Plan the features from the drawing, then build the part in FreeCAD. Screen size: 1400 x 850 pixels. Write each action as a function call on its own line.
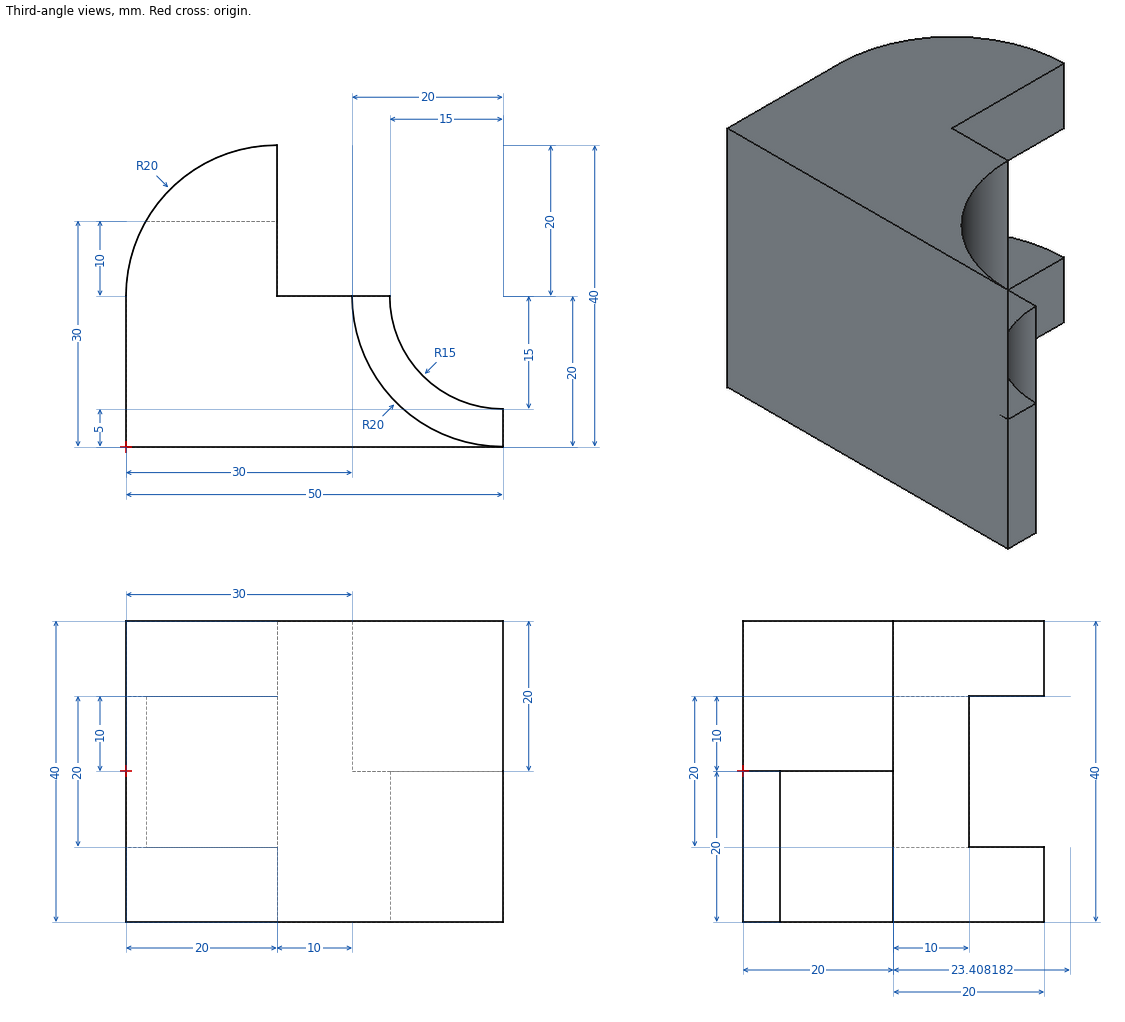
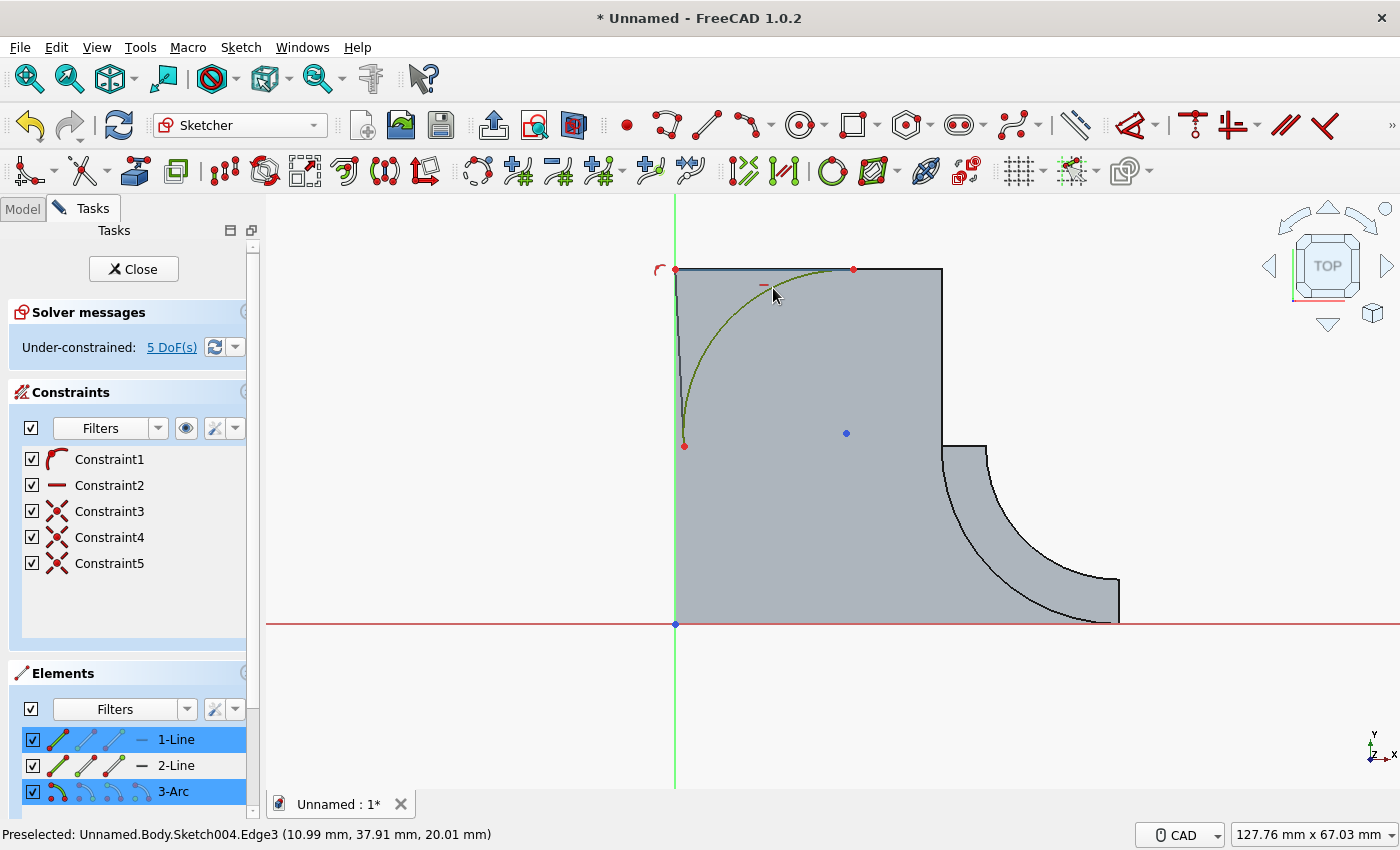
key(t)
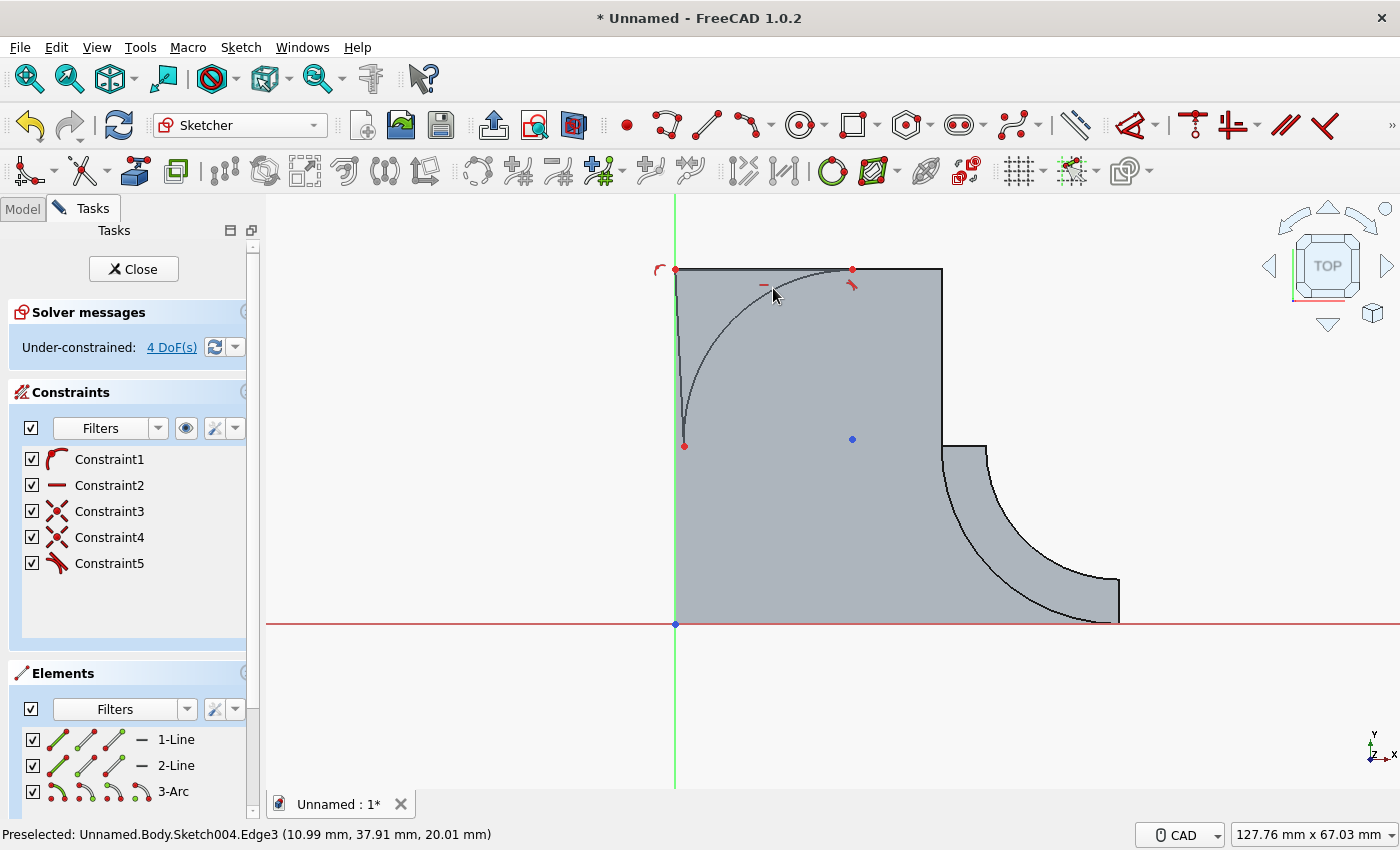
click(678, 323)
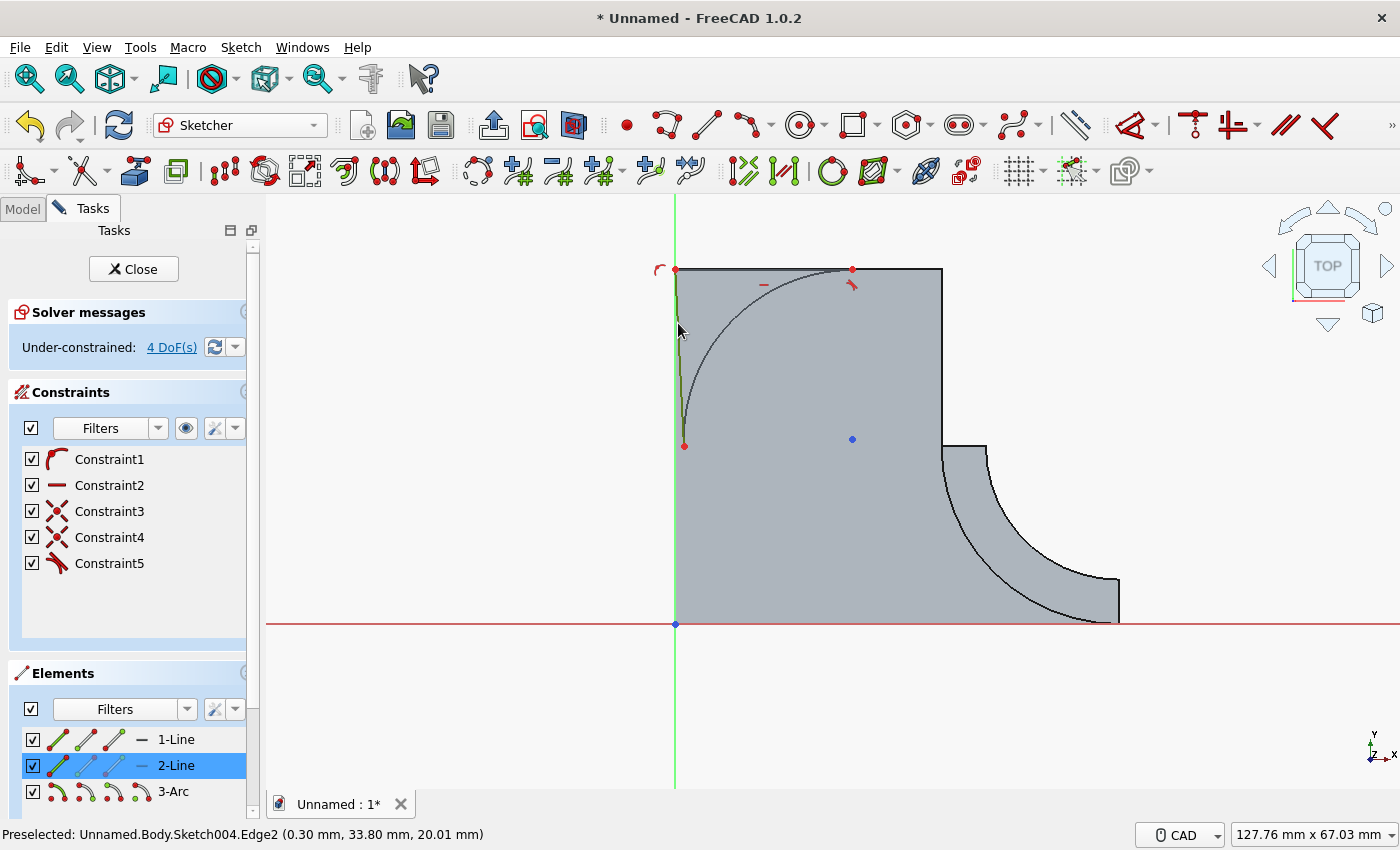
click(774, 290)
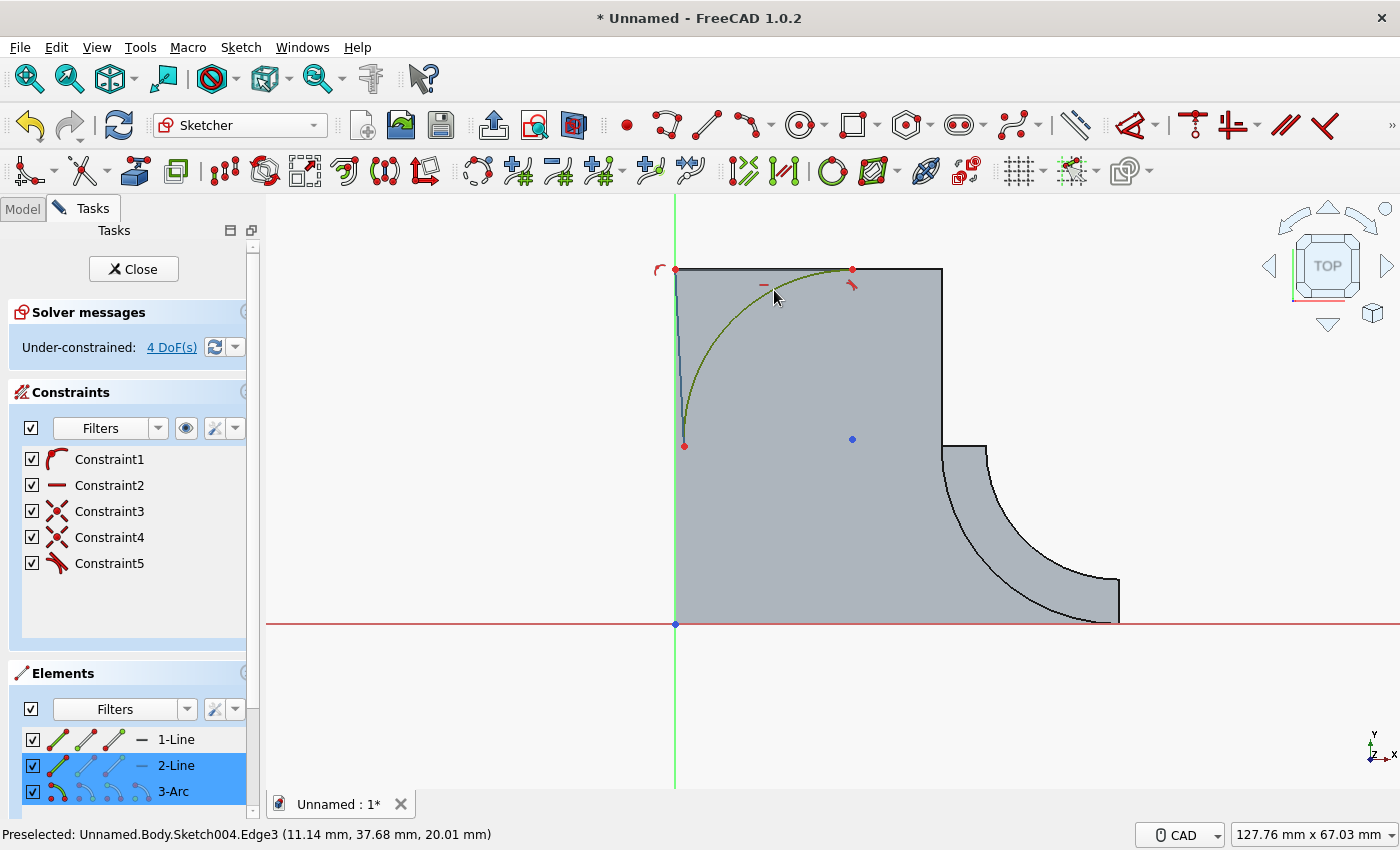
key(t)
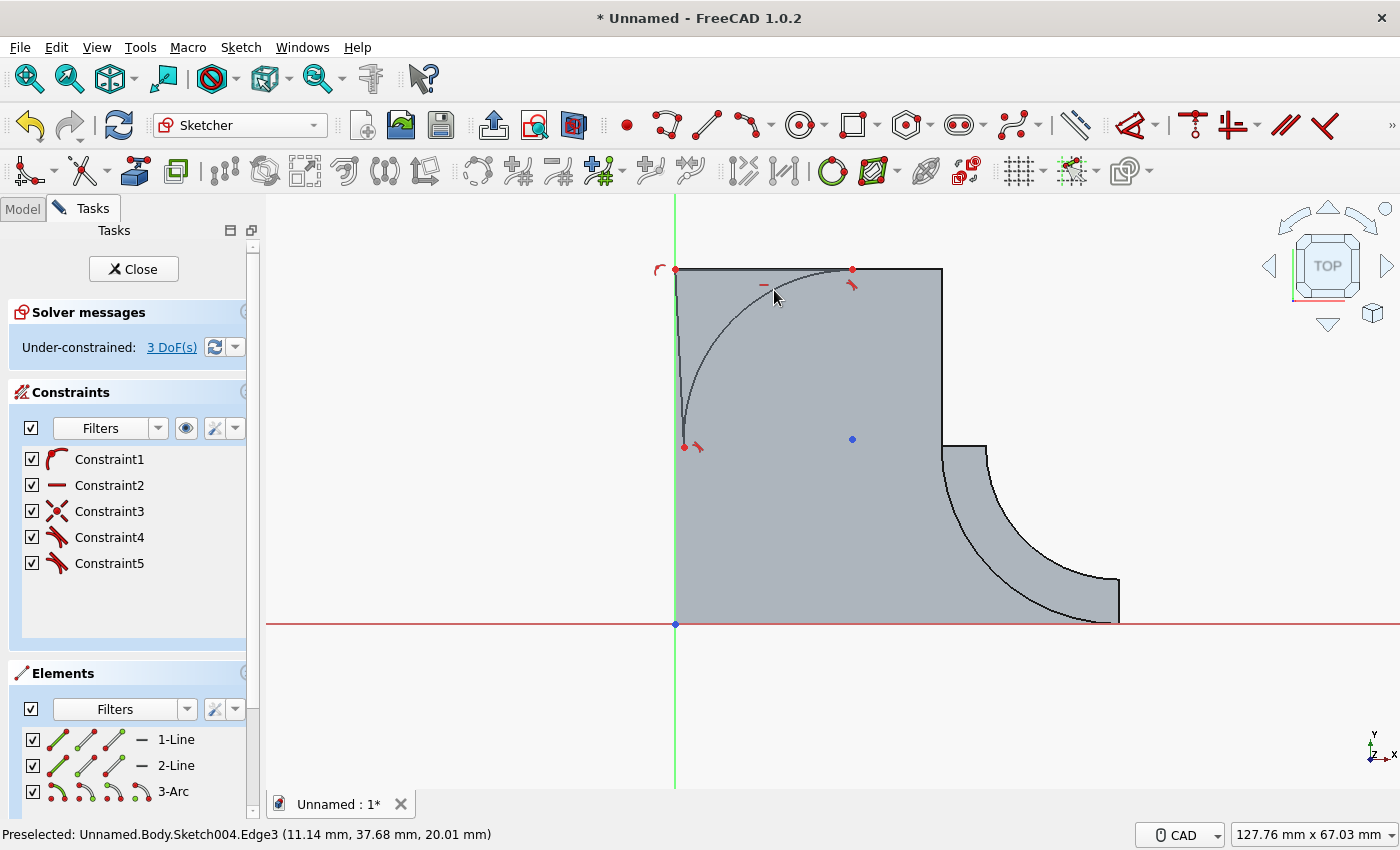
click(678, 323)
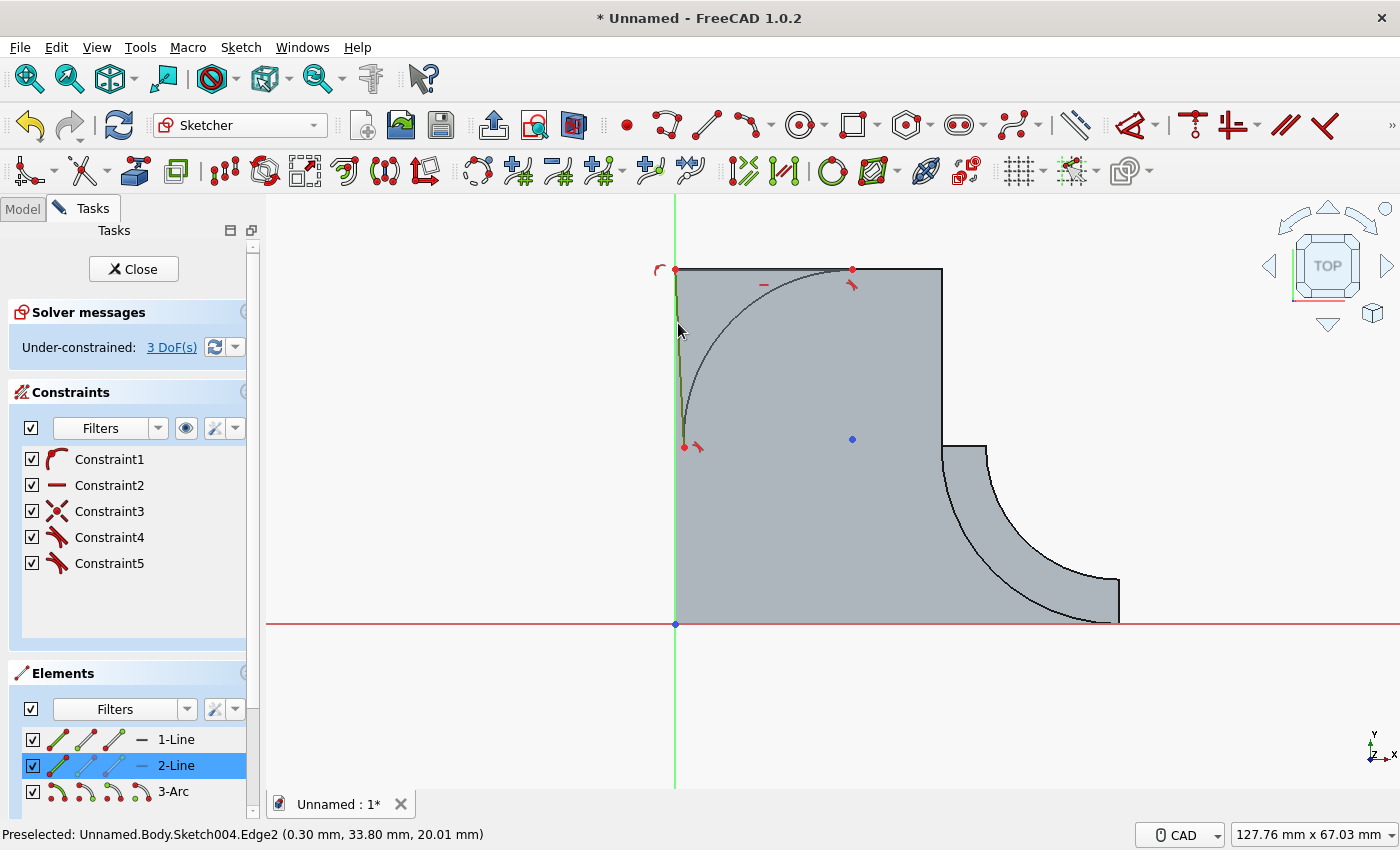
key(v)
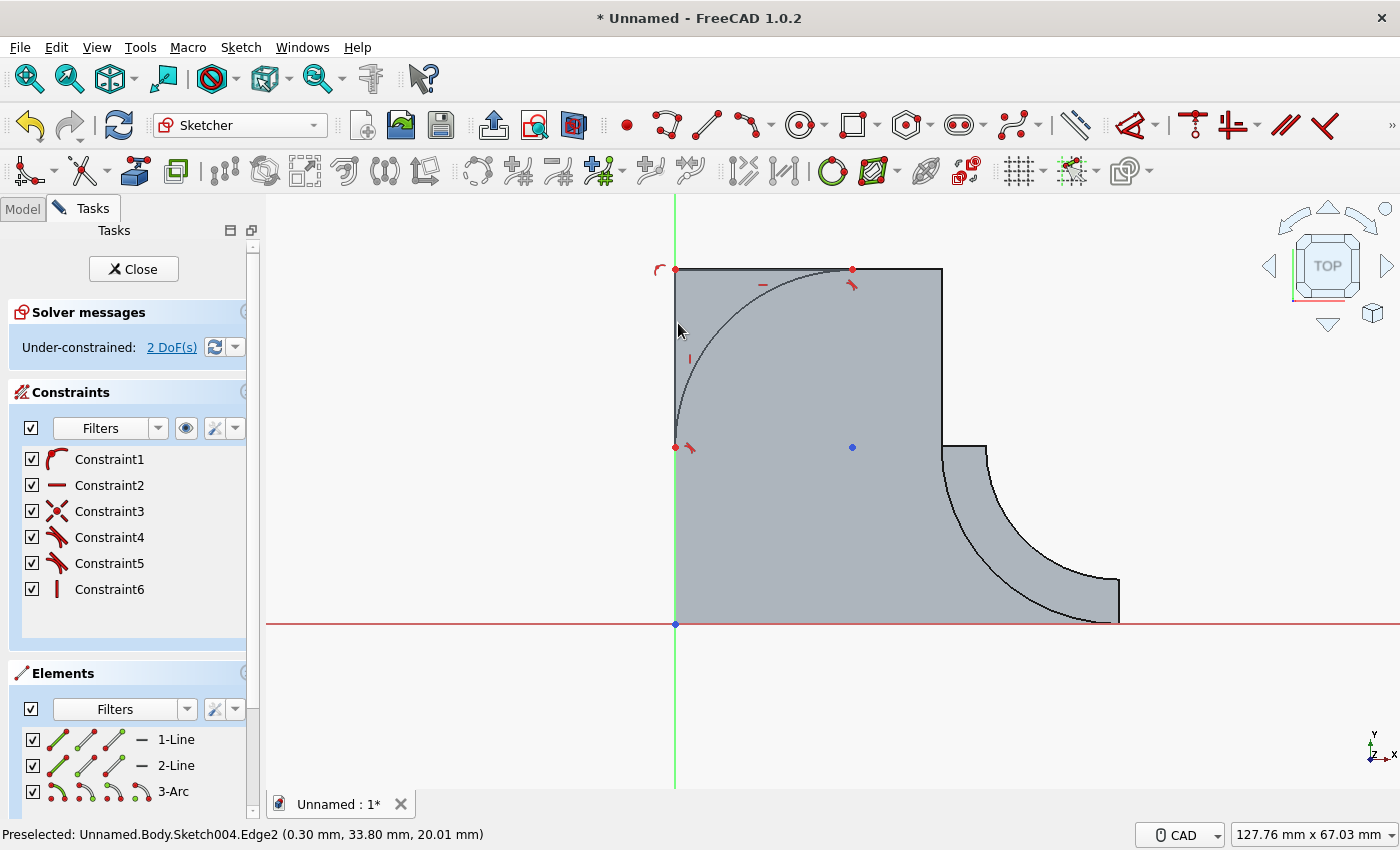
click(1130, 126)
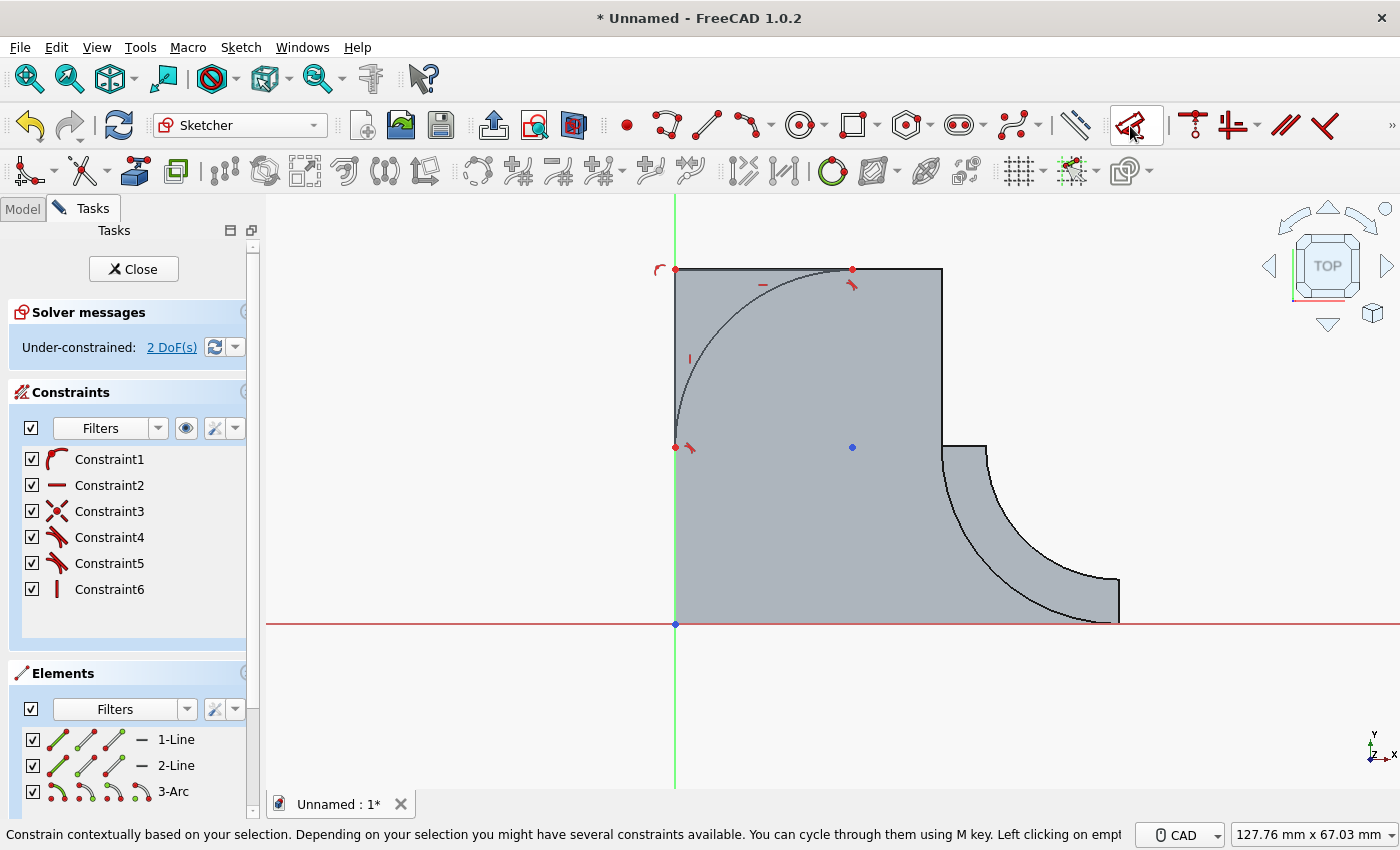
click(772, 289)
click(859, 238)